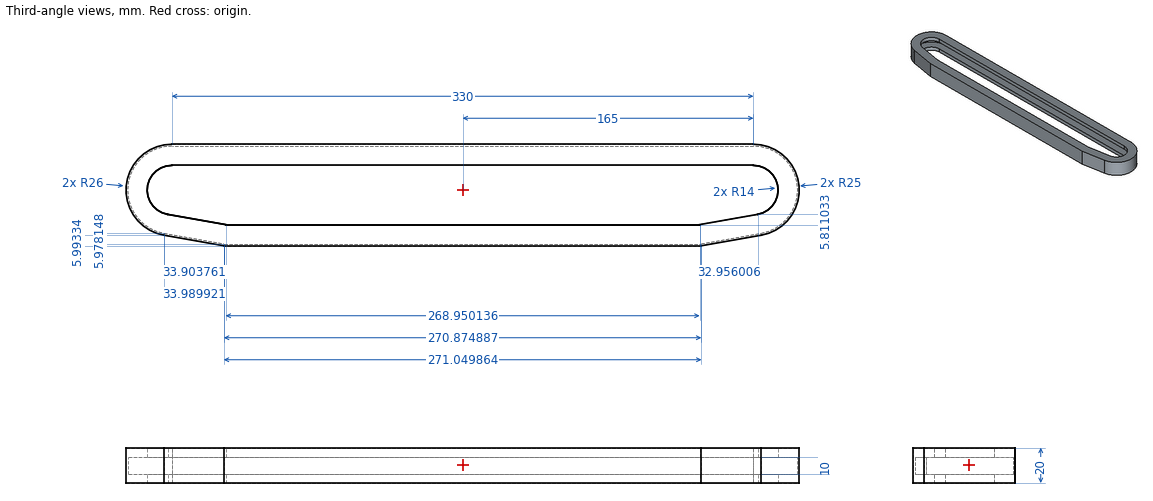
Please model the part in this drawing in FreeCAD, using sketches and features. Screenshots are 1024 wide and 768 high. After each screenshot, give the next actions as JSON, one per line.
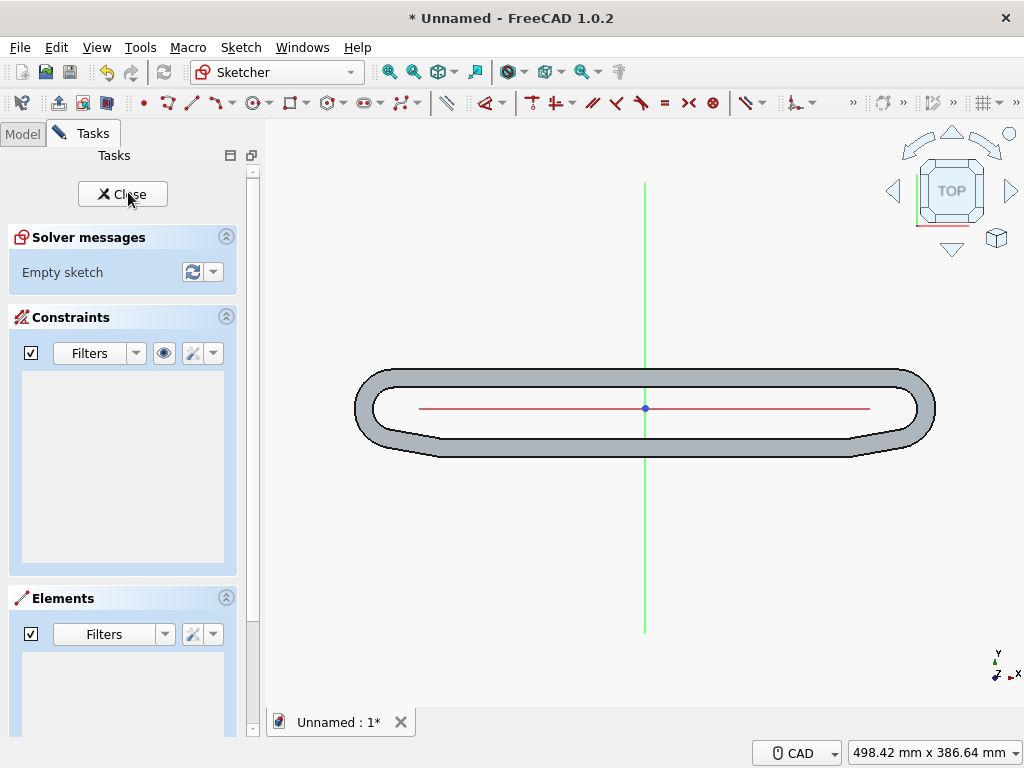
{"action": "left_click", "coordinate": [108, 104]}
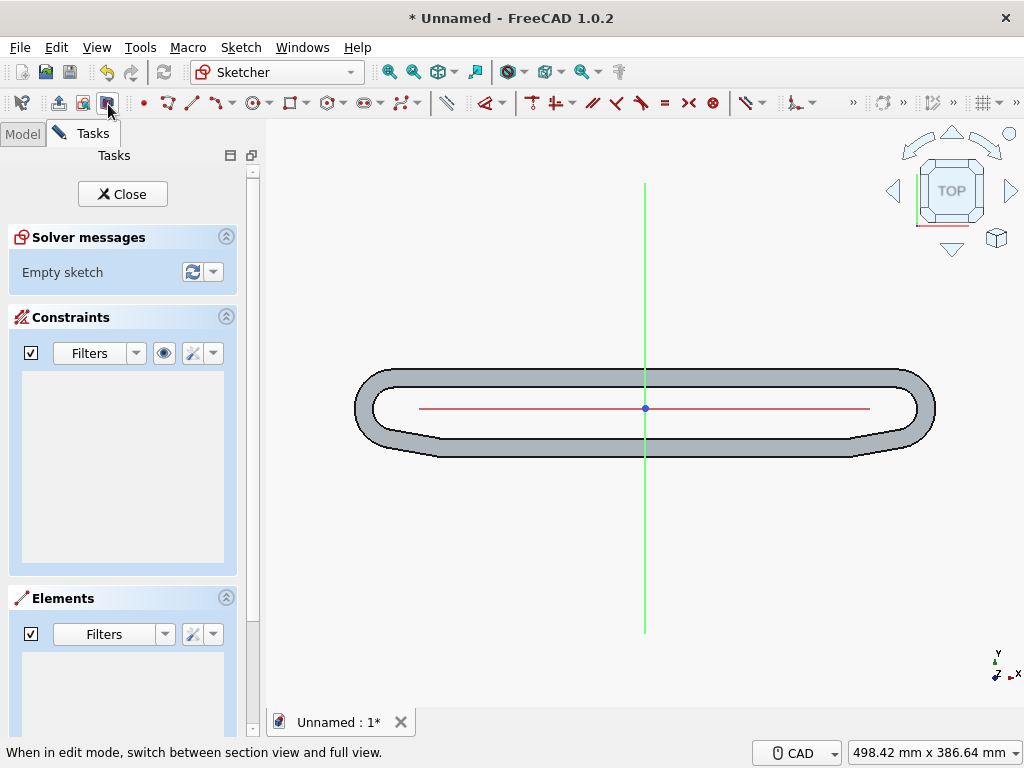
{"action": "scroll", "coordinate": [437, 413], "scroll_direction": "down", "scroll_amount": 2}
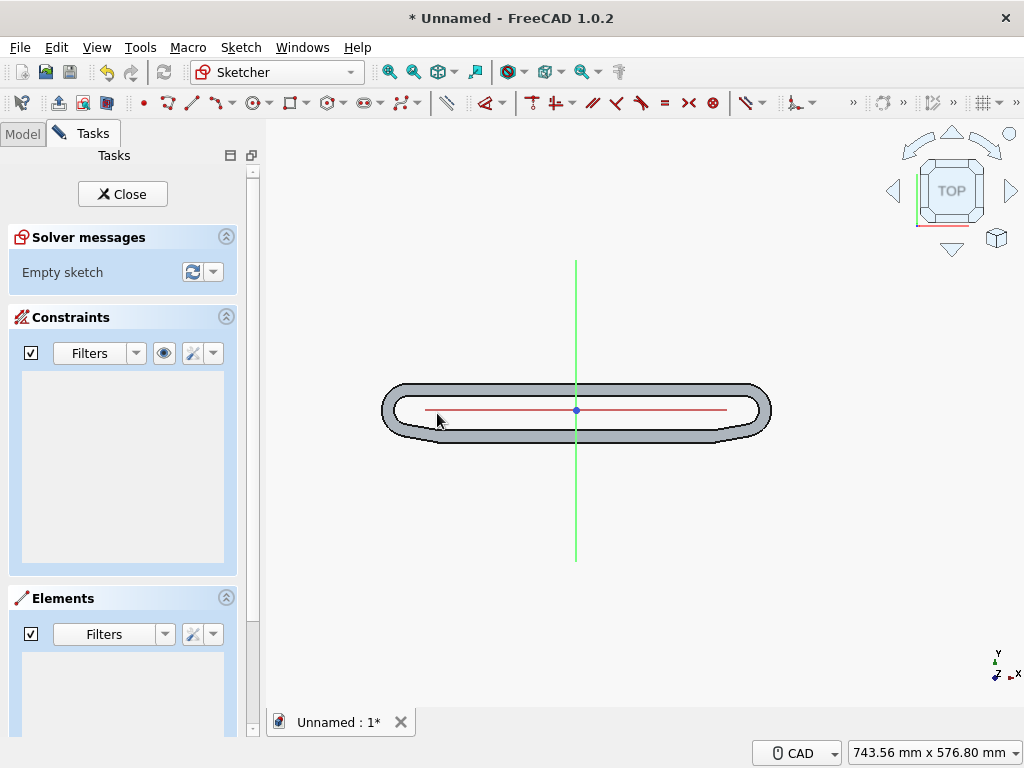
{"action": "left_click", "coordinate": [192, 104]}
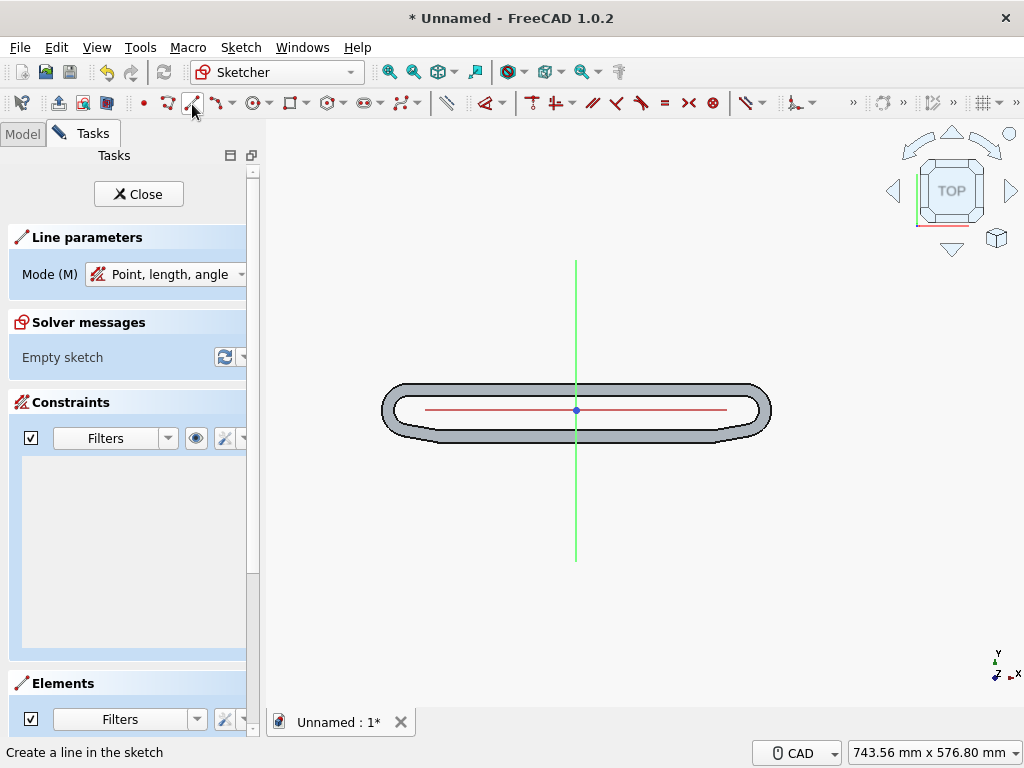
{"action": "left_click", "coordinate": [745, 385]}
{"action": "left_click", "coordinate": [408, 385]}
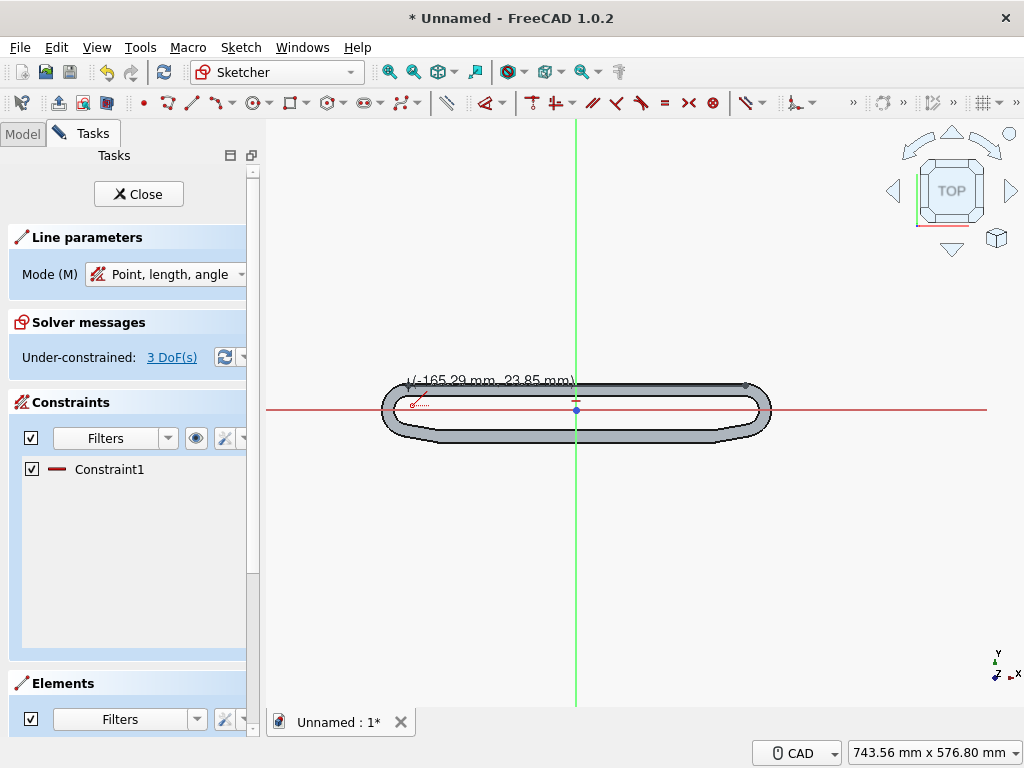
{"action": "left_click", "coordinate": [168, 104]}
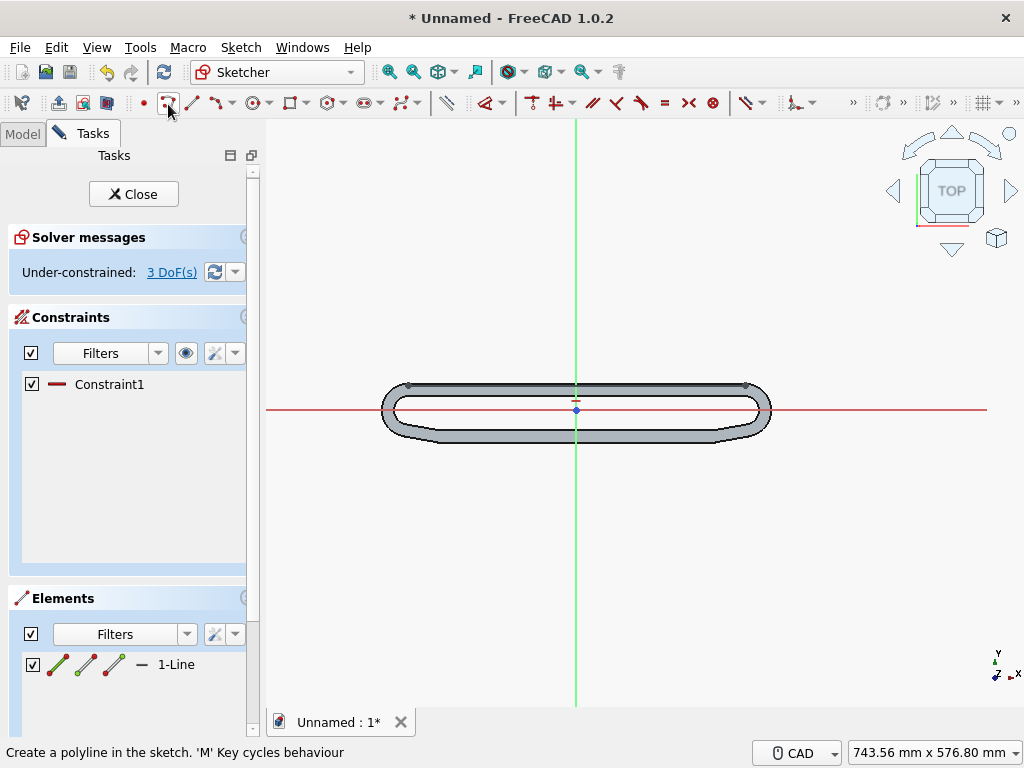
{"action": "left_click", "coordinate": [404, 435]}
{"action": "left_click", "coordinate": [438, 442]}
{"action": "left_click", "coordinate": [715, 442]}
{"action": "left_click", "coordinate": [749, 435]}
{"action": "right_click", "coordinate": [749, 435]}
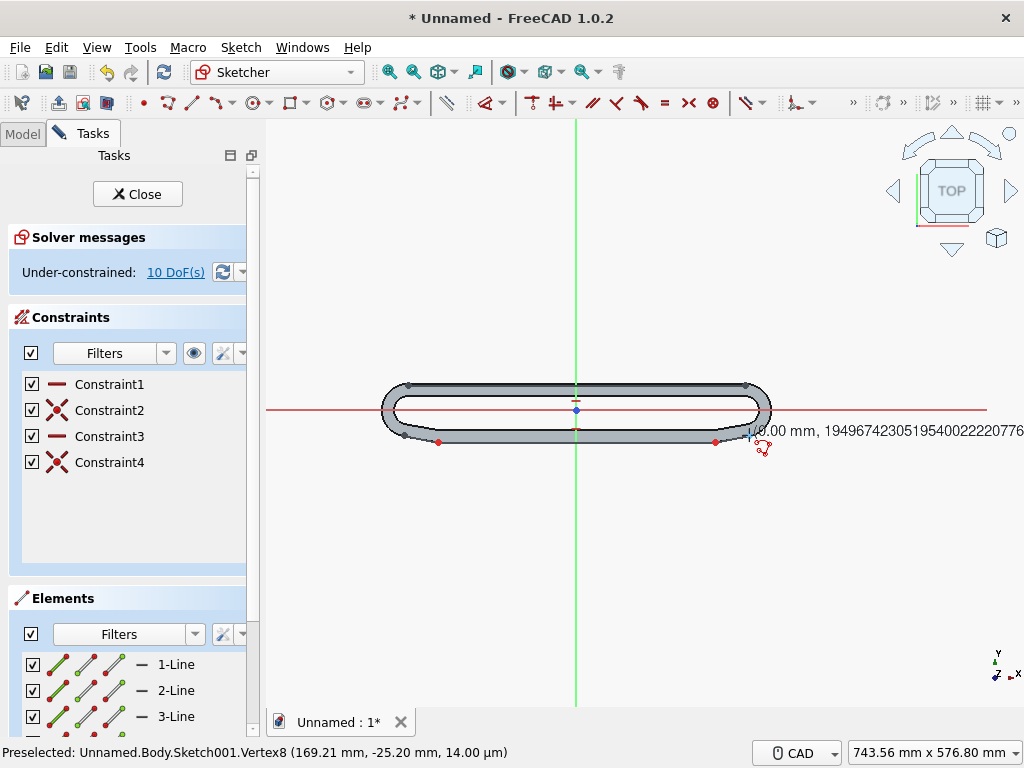
{"action": "left_click", "coordinate": [216, 104]}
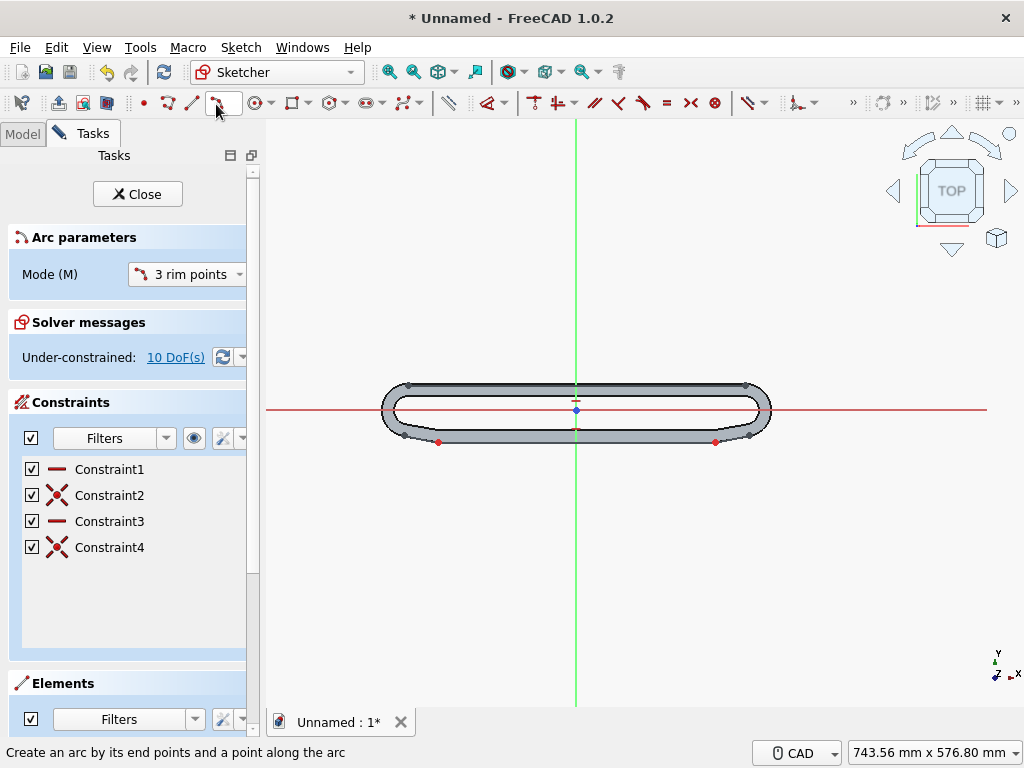
{"action": "left_click", "coordinate": [408, 386]}
{"action": "left_click", "coordinate": [404, 436]}
{"action": "left_click", "coordinate": [388, 394]}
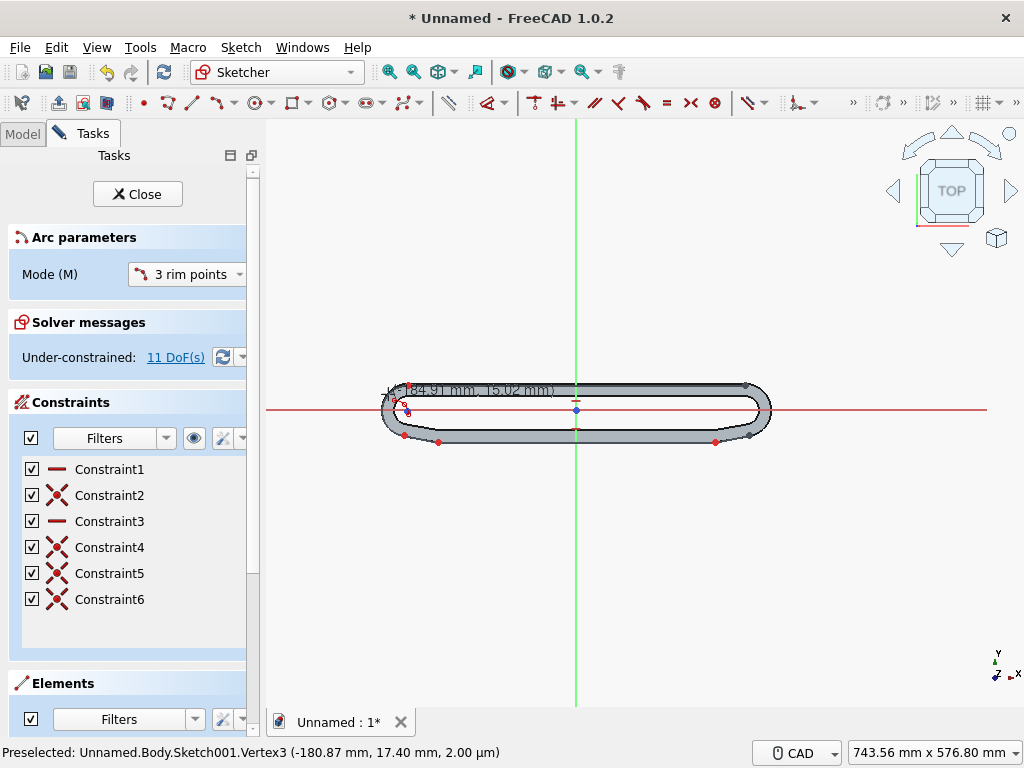
{"action": "left_click", "coordinate": [749, 436]}
{"action": "left_click", "coordinate": [745, 386]}
{"action": "left_click", "coordinate": [765, 394]}
{"action": "key", "text": "Escape"}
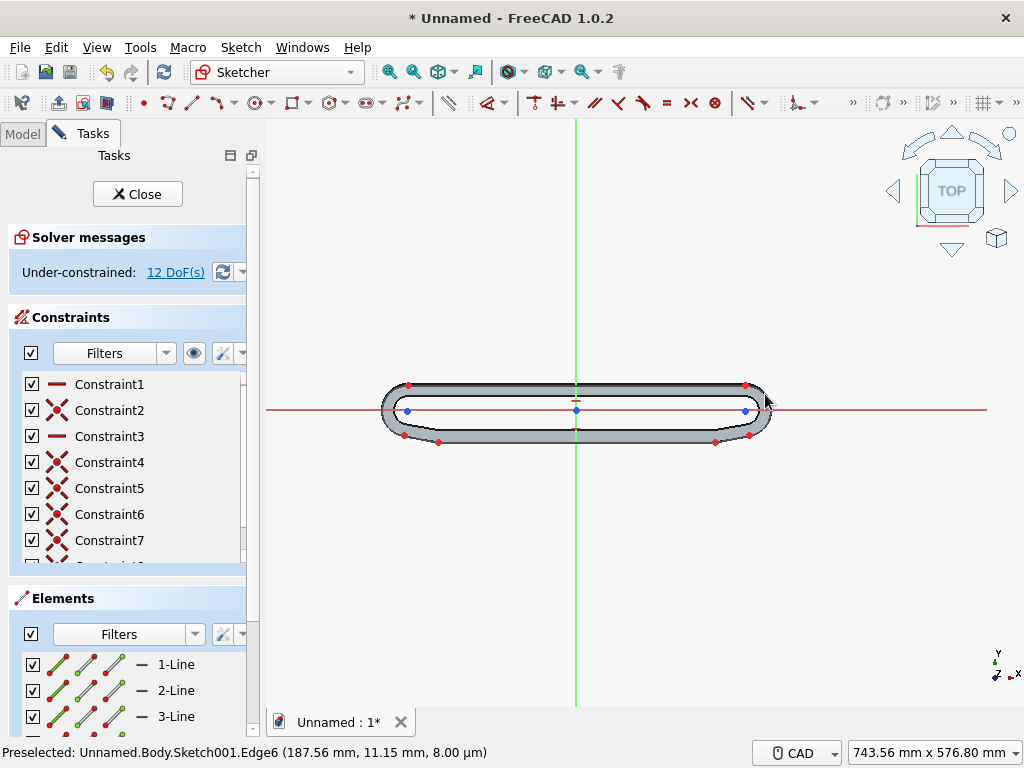
{"action": "left_click", "coordinate": [644, 386]}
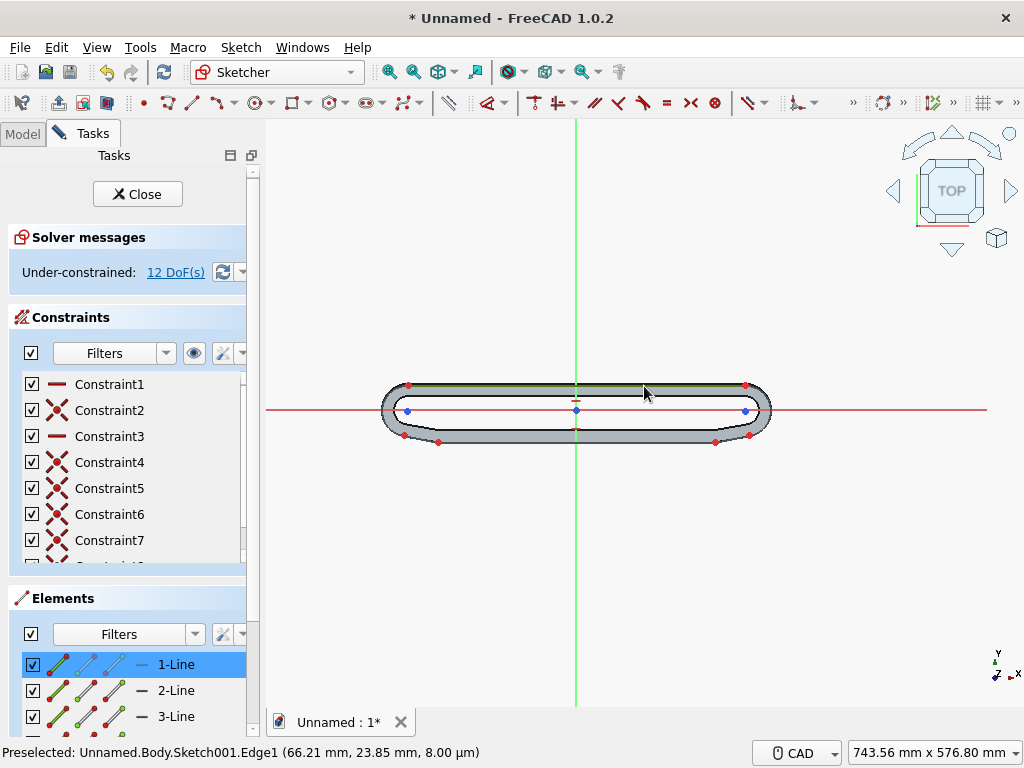
{"action": "left_click", "coordinate": [388, 395]}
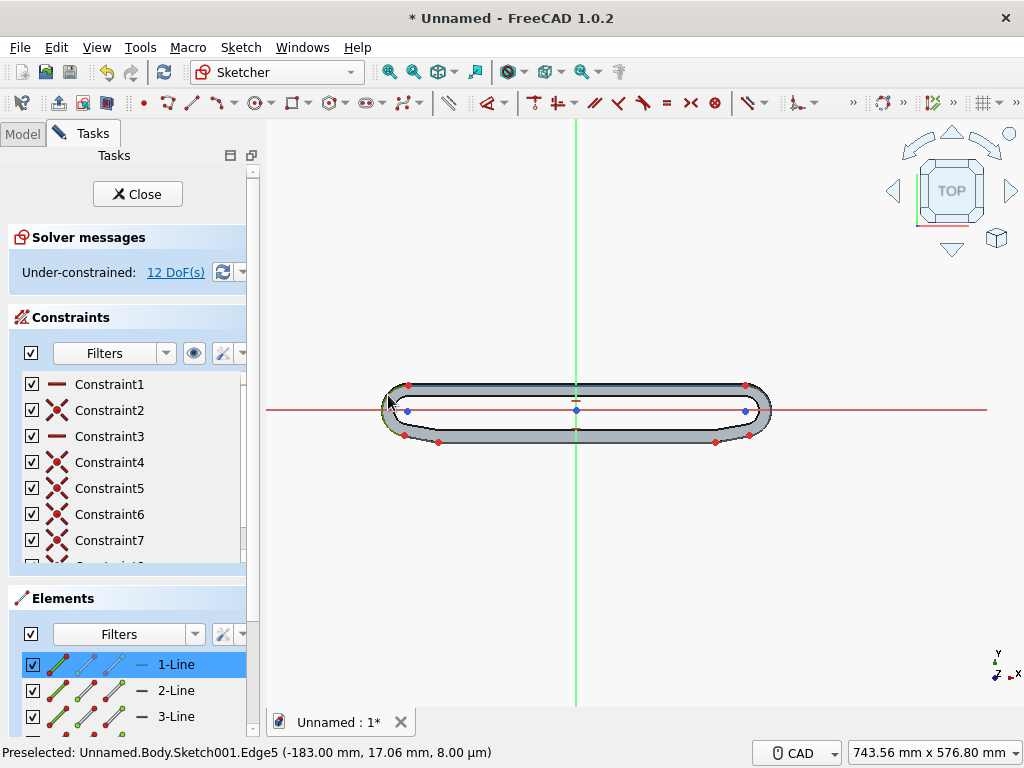
{"action": "left_click", "coordinate": [644, 104]}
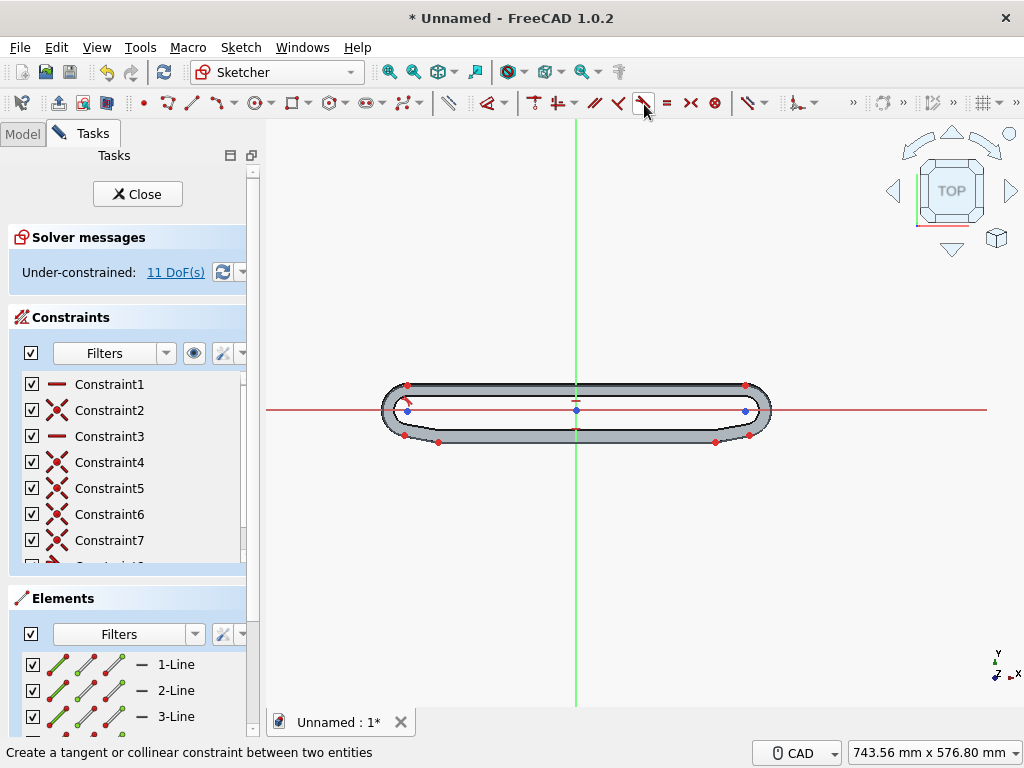
{"action": "left_click", "coordinate": [644, 386]}